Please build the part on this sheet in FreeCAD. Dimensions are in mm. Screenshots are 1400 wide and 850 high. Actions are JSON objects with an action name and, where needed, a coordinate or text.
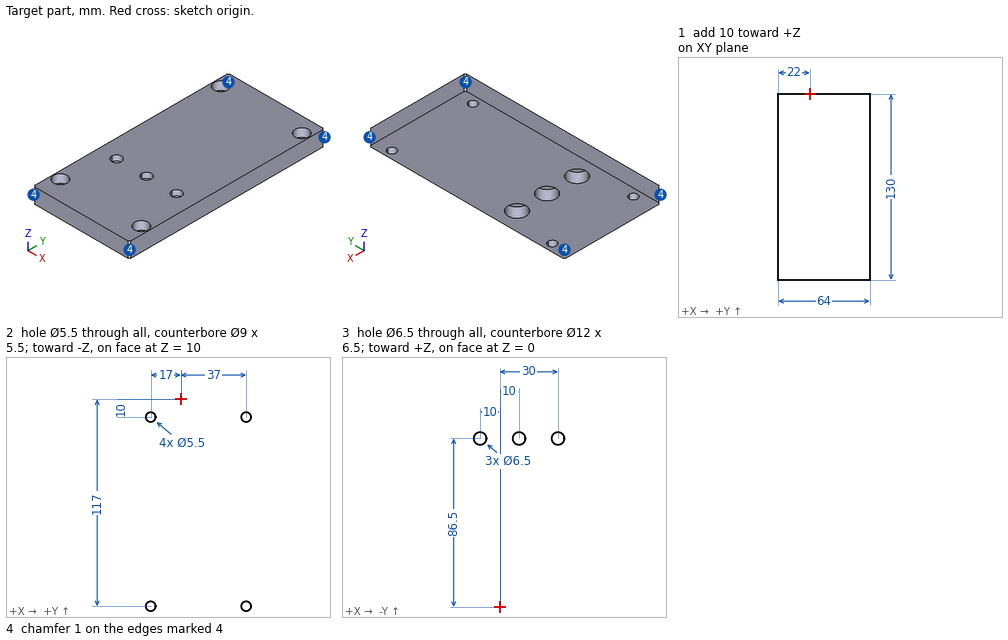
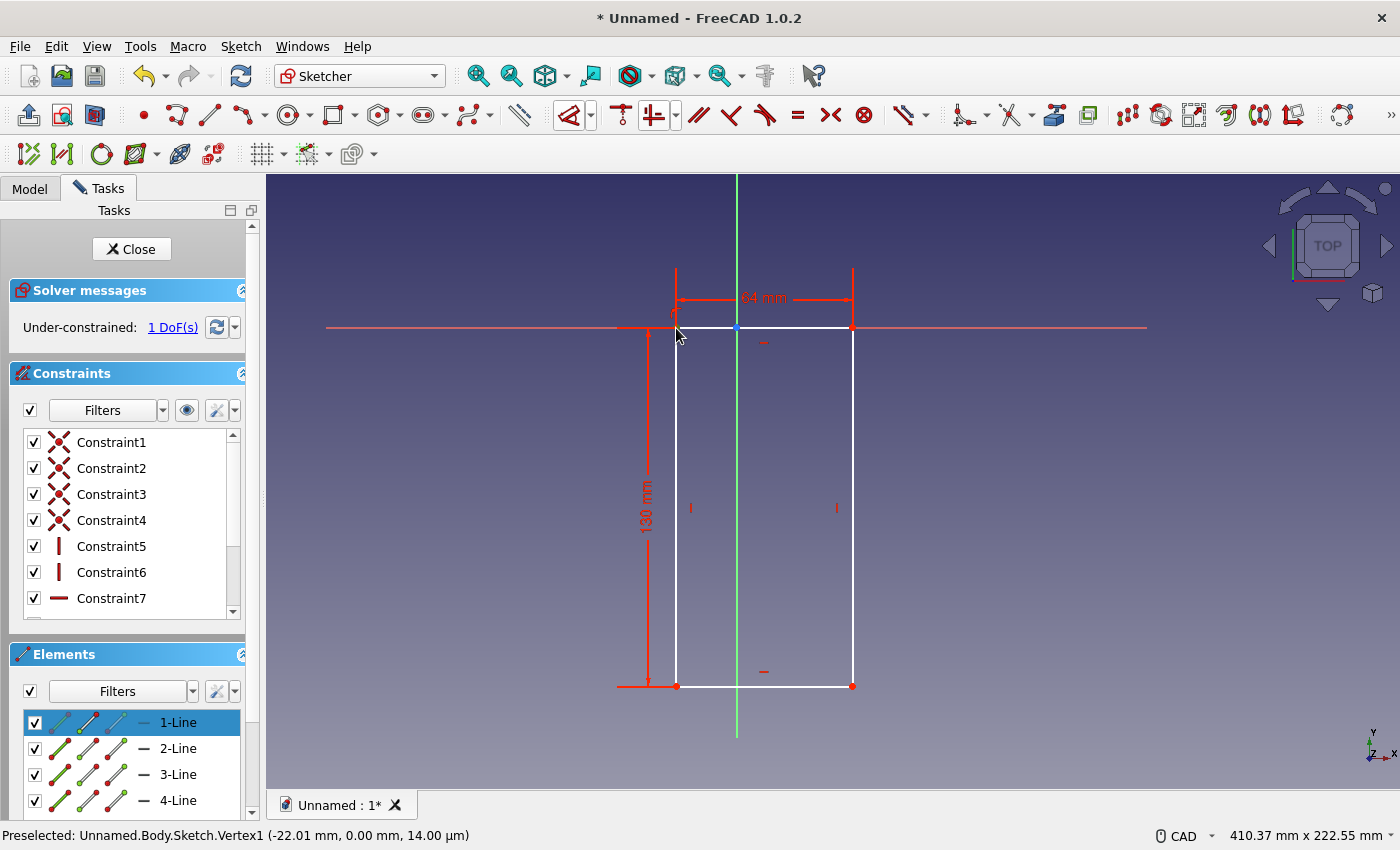
{"action": "key", "text": "l"}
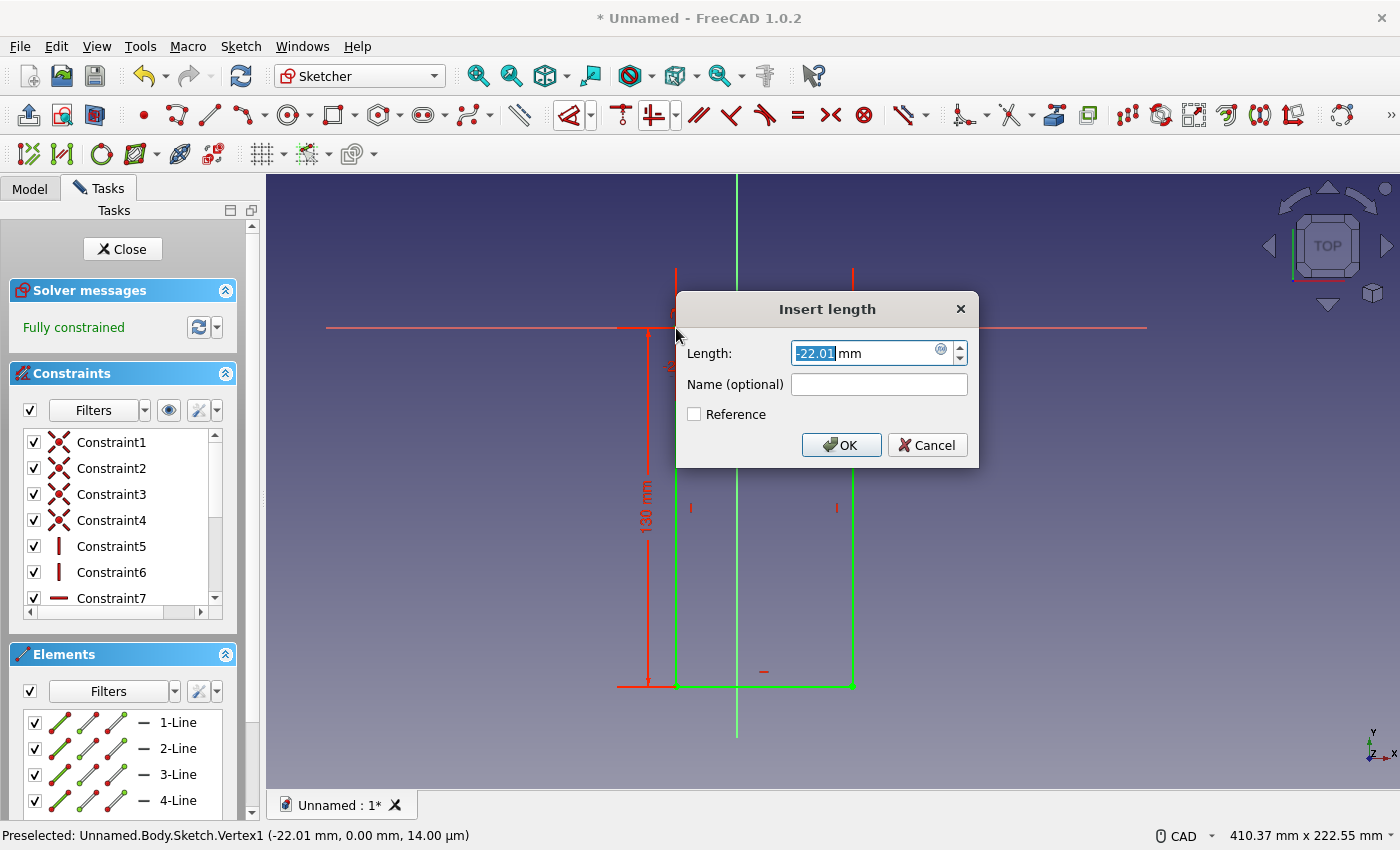
{"action": "type", "text": "-22"}
{"action": "key", "text": "Return"}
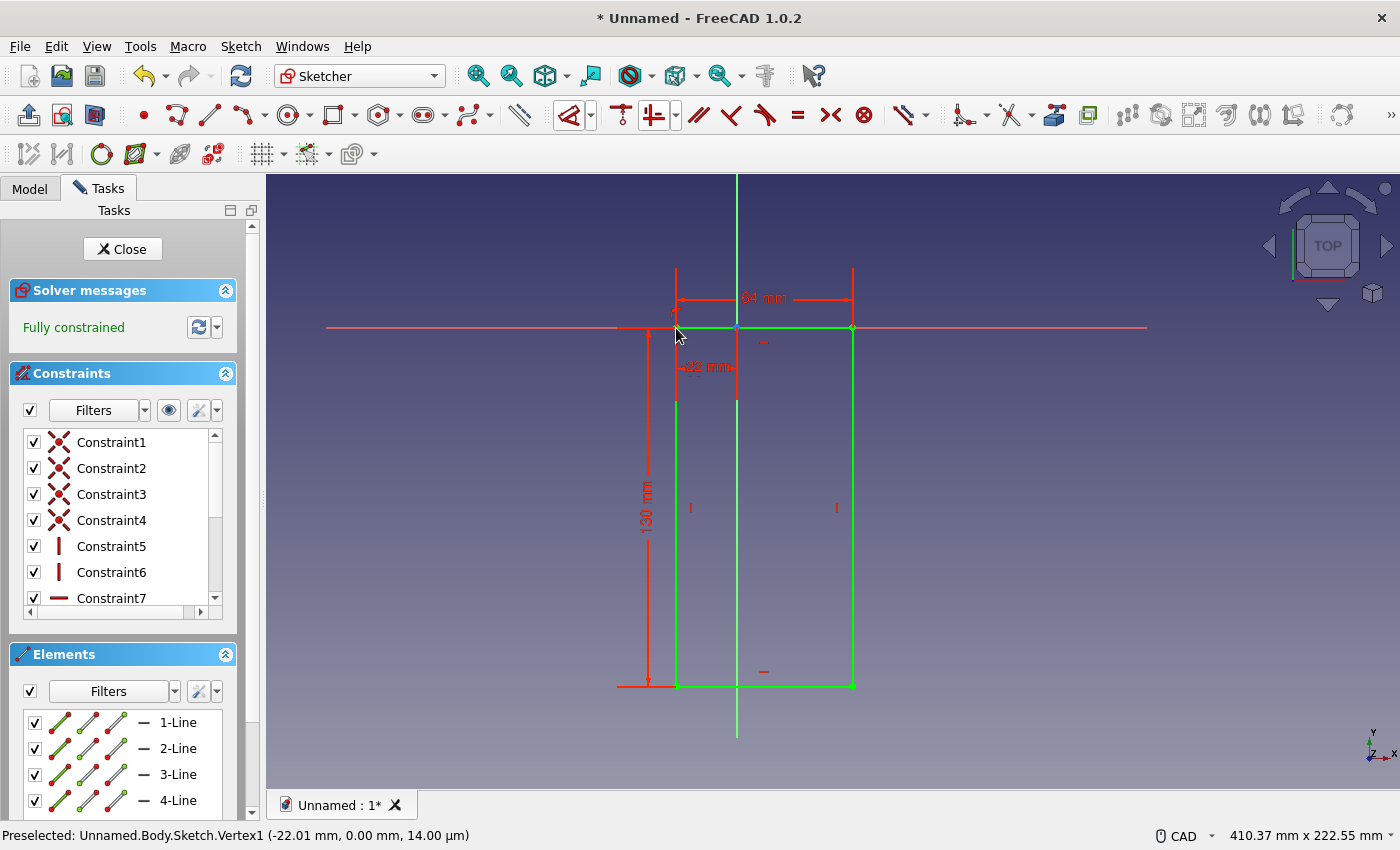
{"action": "left_click", "coordinate": [123, 249]}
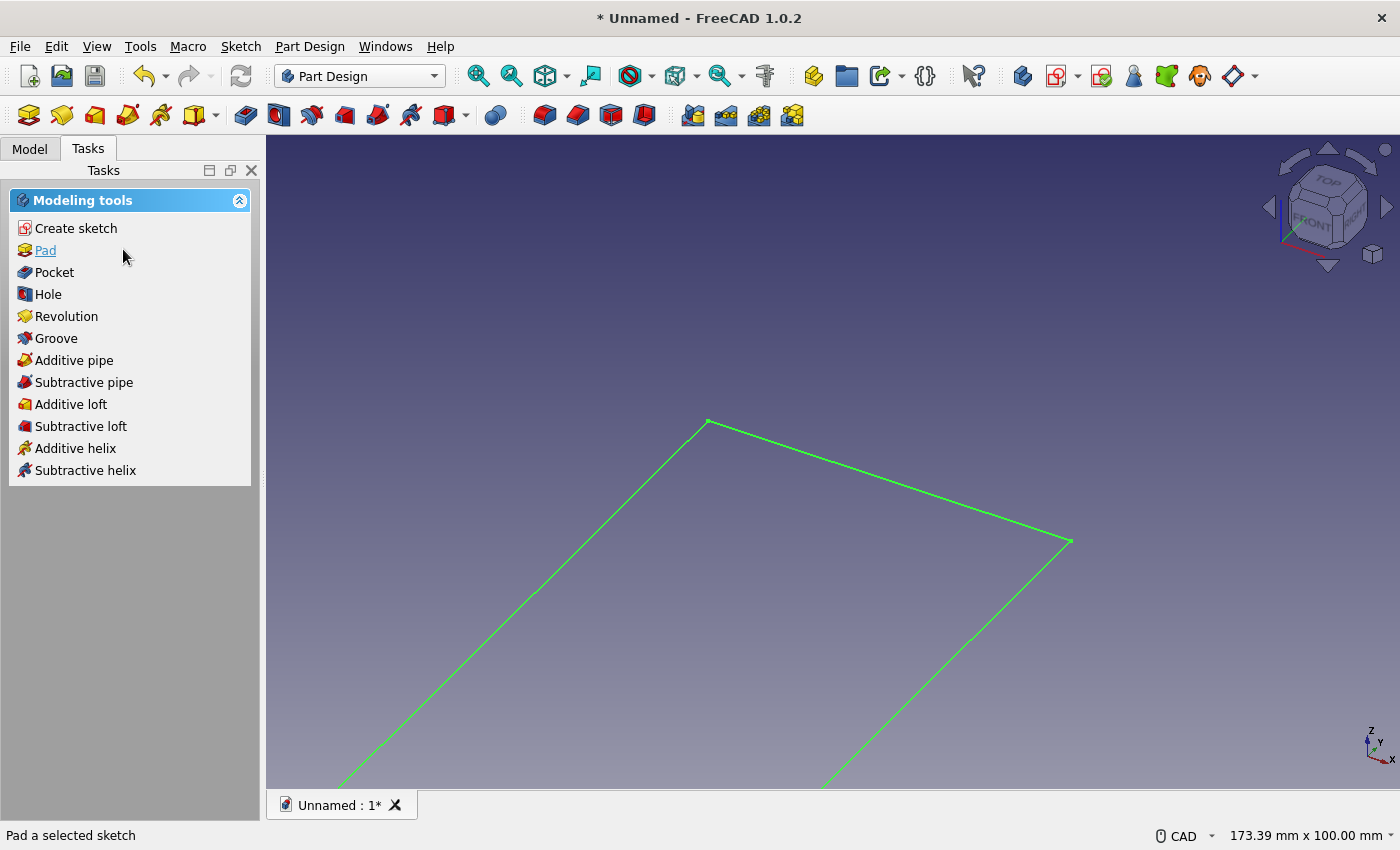
{"action": "left_click", "coordinate": [29, 116]}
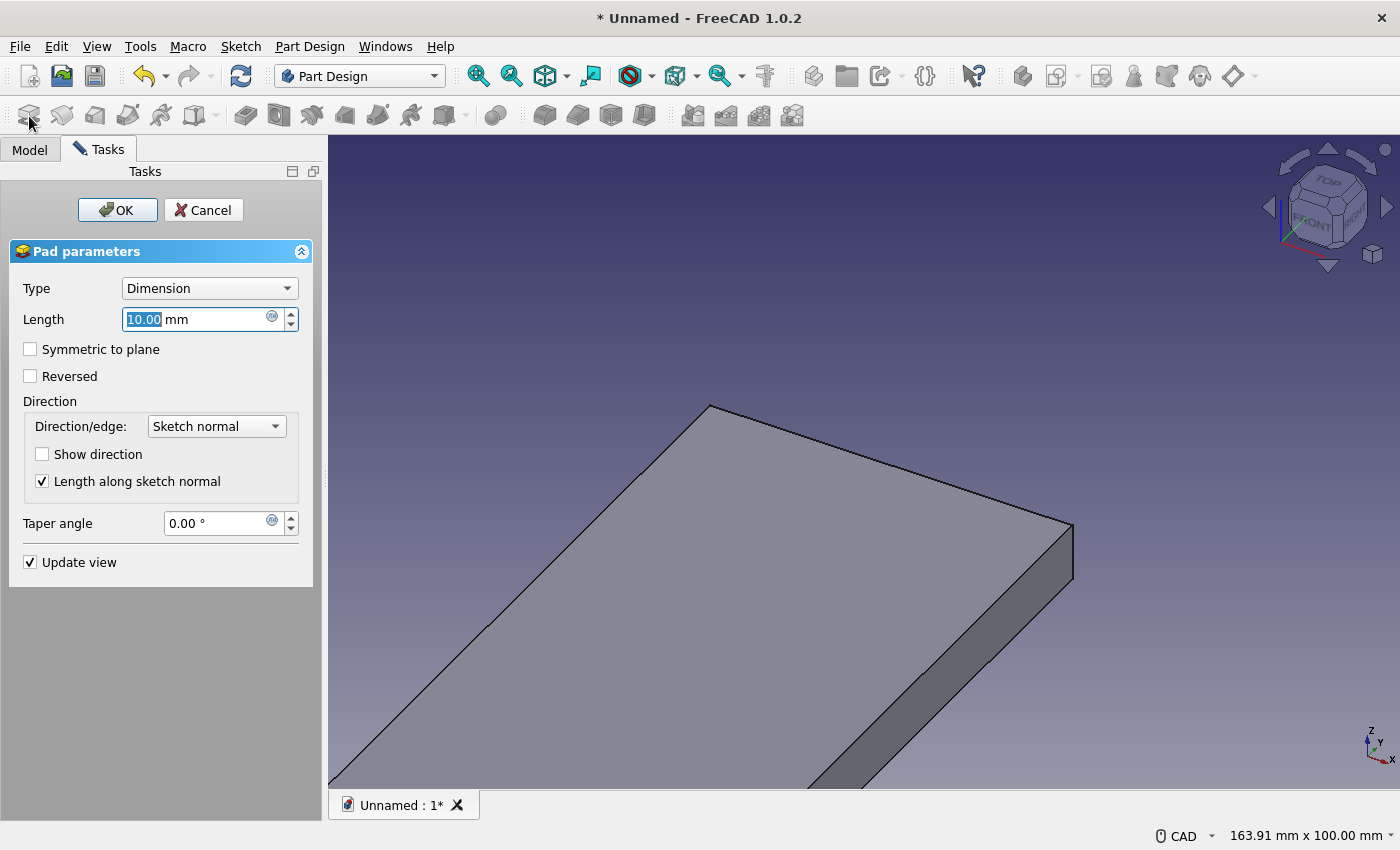
{"action": "type", "text": "10"}
{"action": "key", "text": "Tab"}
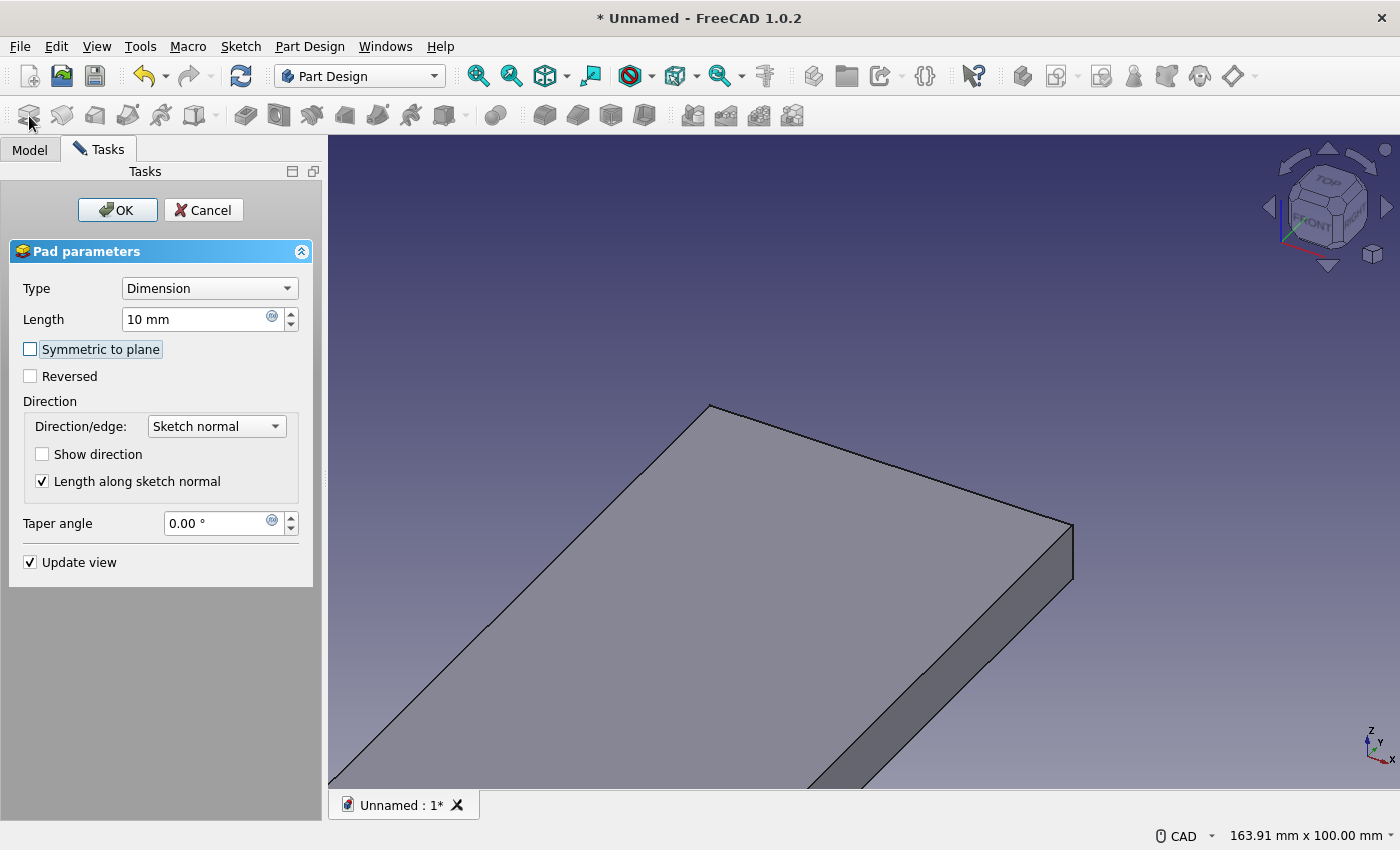
{"action": "left_click", "coordinate": [118, 210]}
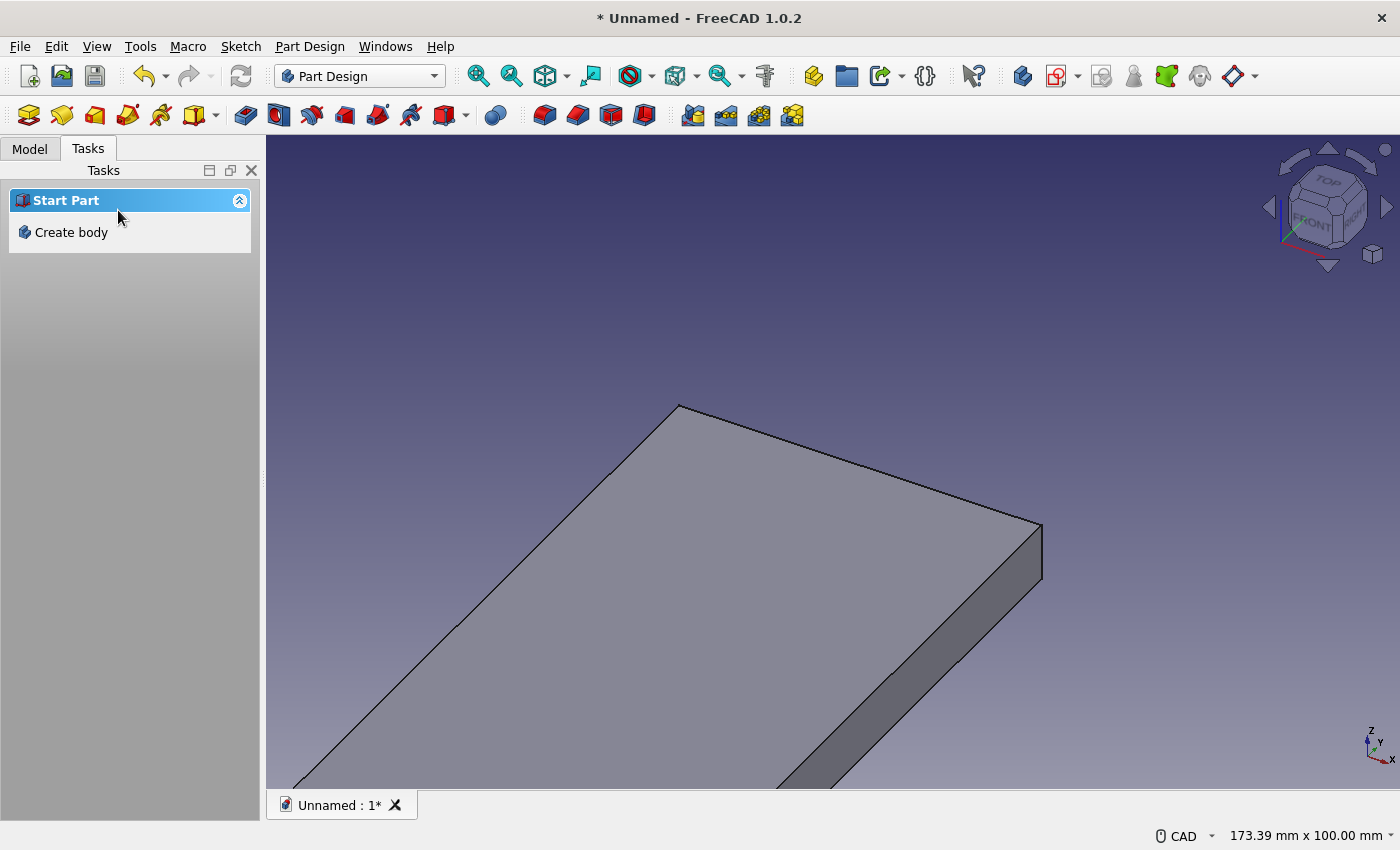
{"action": "key", "text": "v f"}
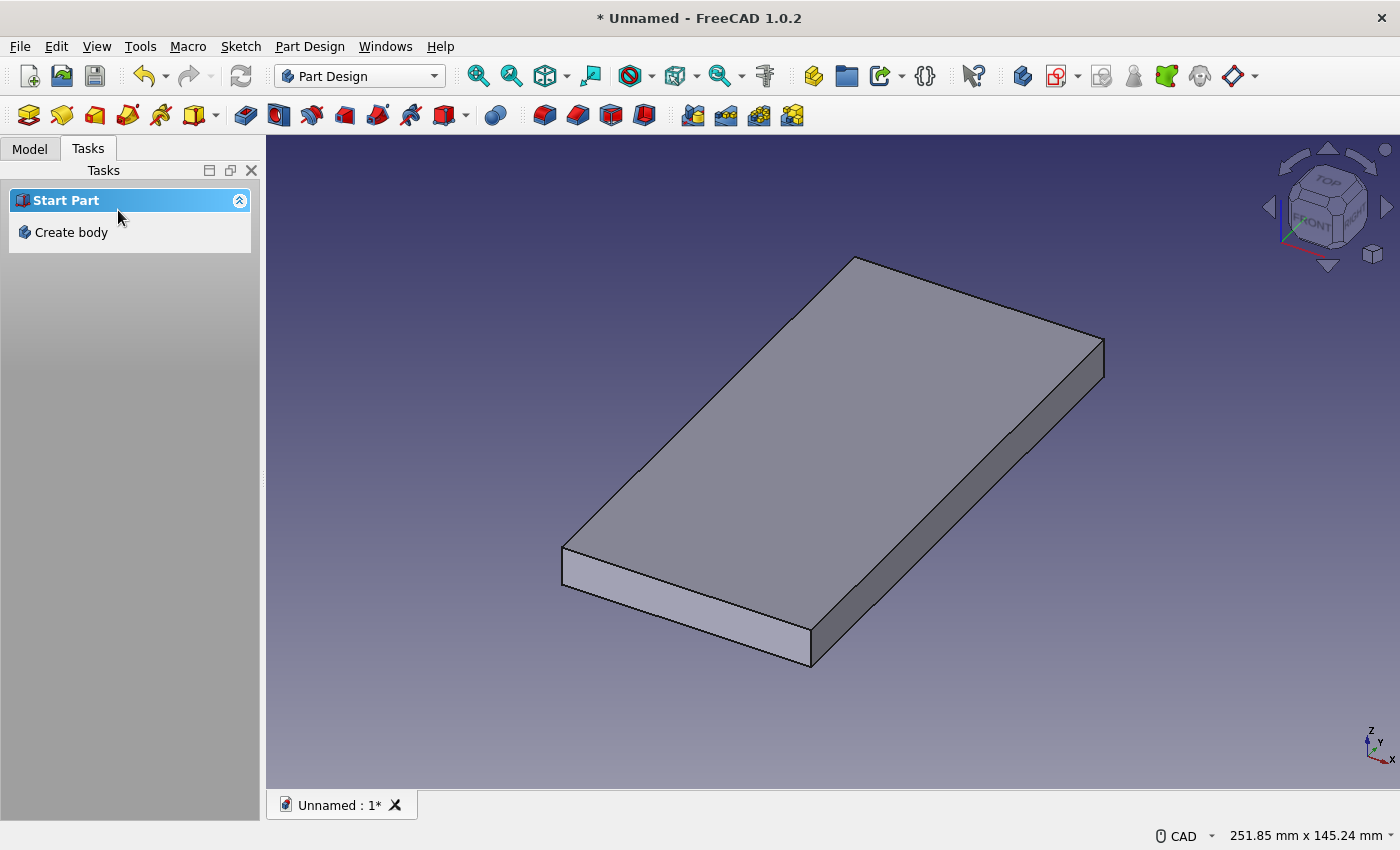
{"action": "left_click", "coordinate": [875, 401]}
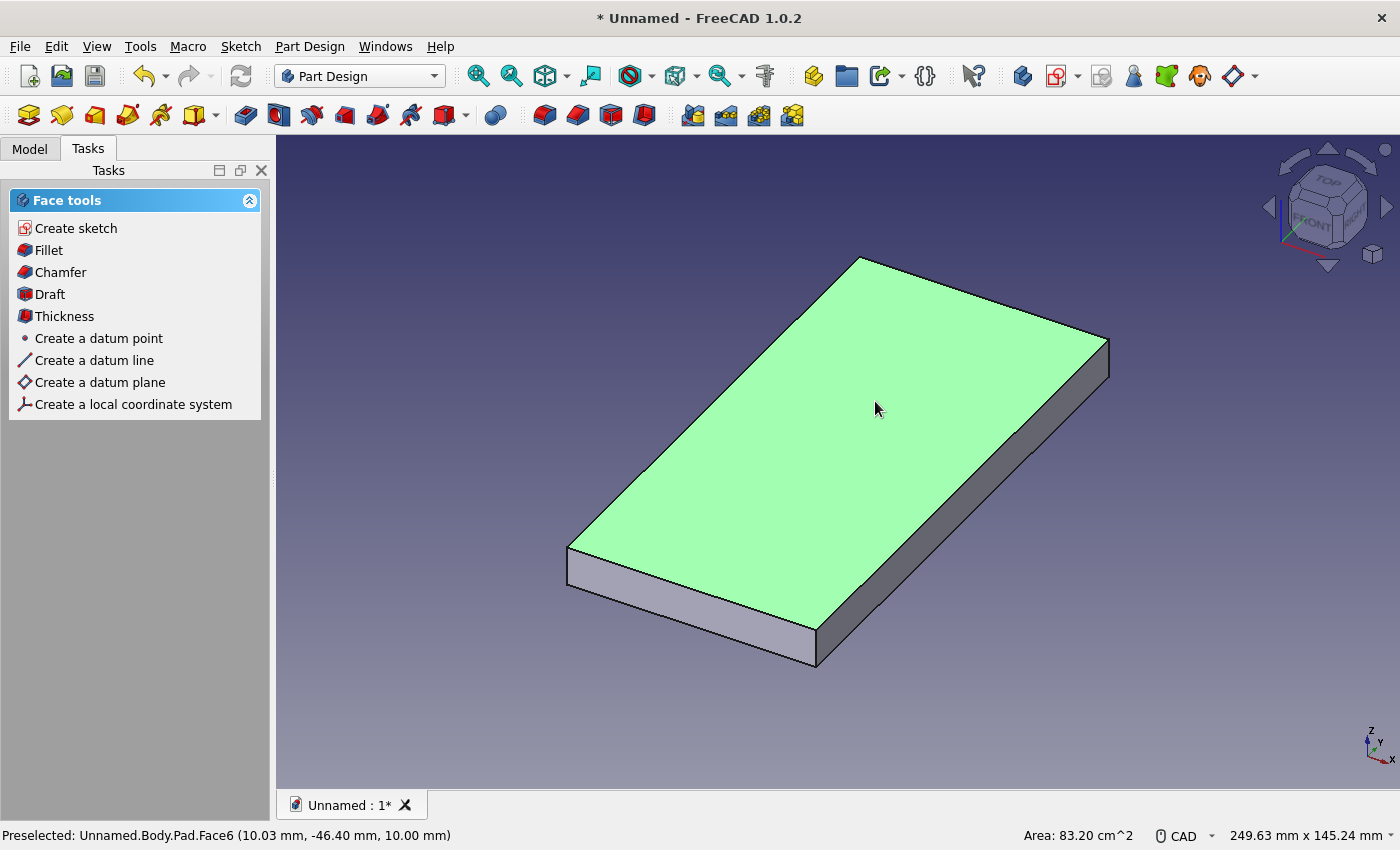
{"action": "left_click", "coordinate": [1056, 76]}